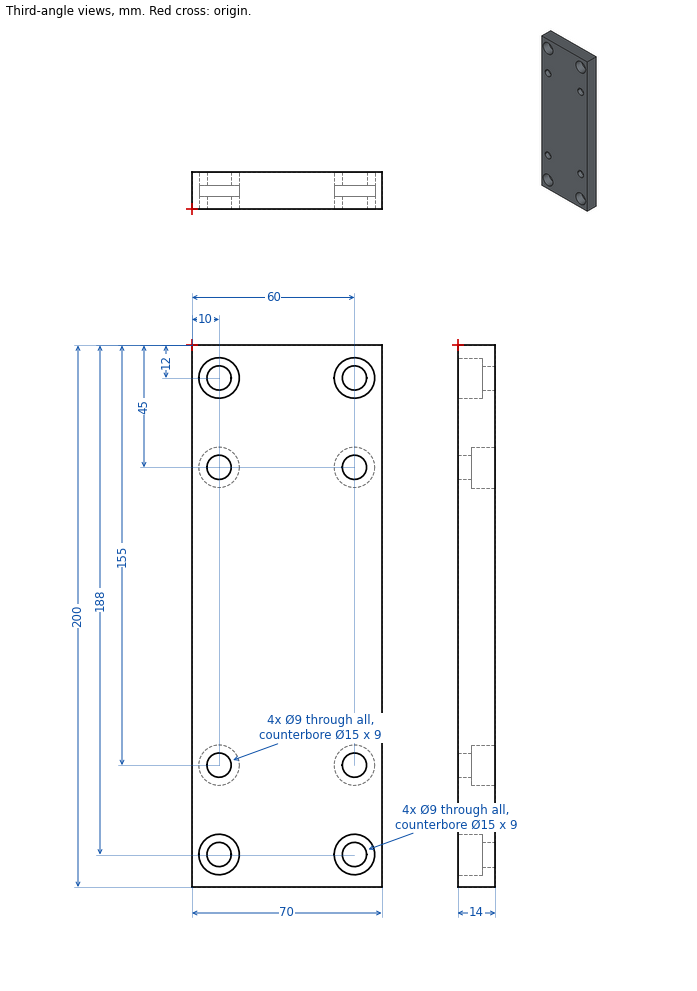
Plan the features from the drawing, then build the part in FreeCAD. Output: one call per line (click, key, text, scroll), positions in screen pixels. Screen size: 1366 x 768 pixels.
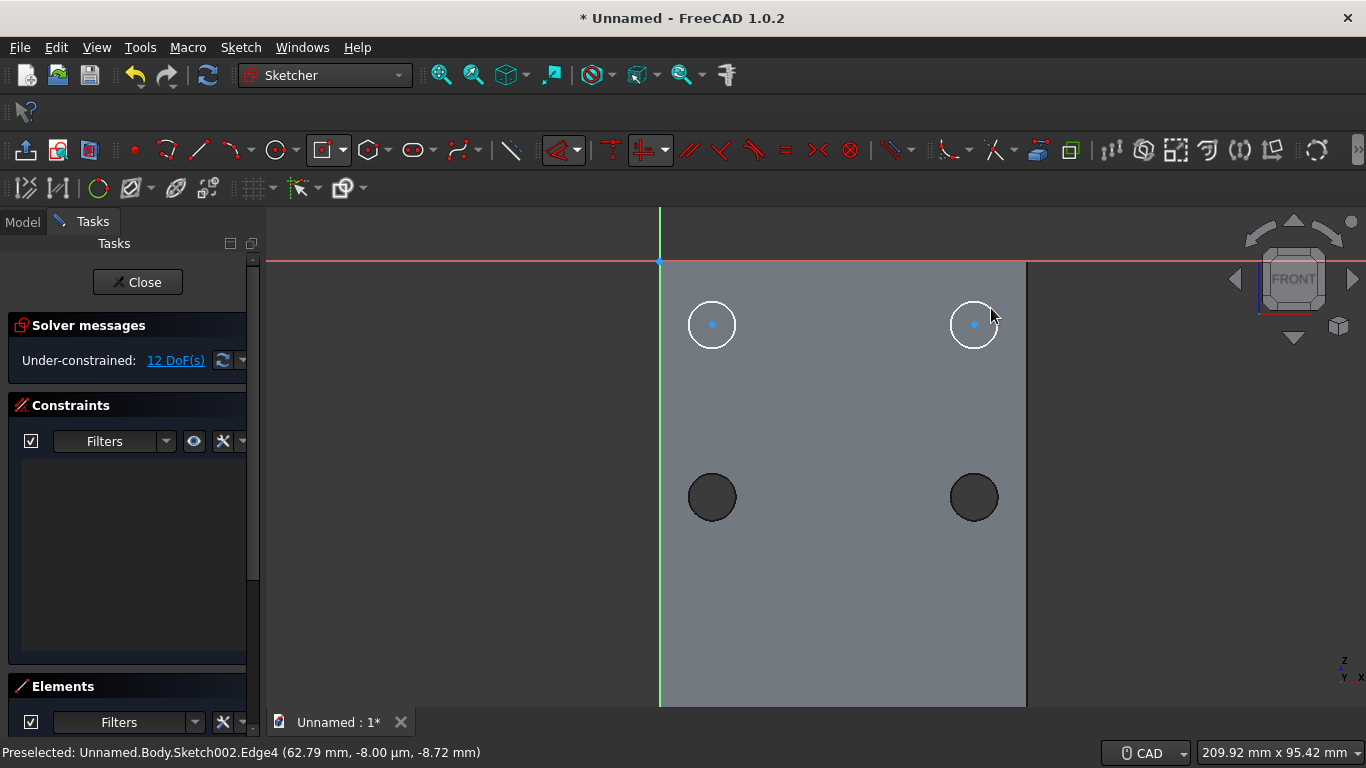
scroll(712, 324, down, 6)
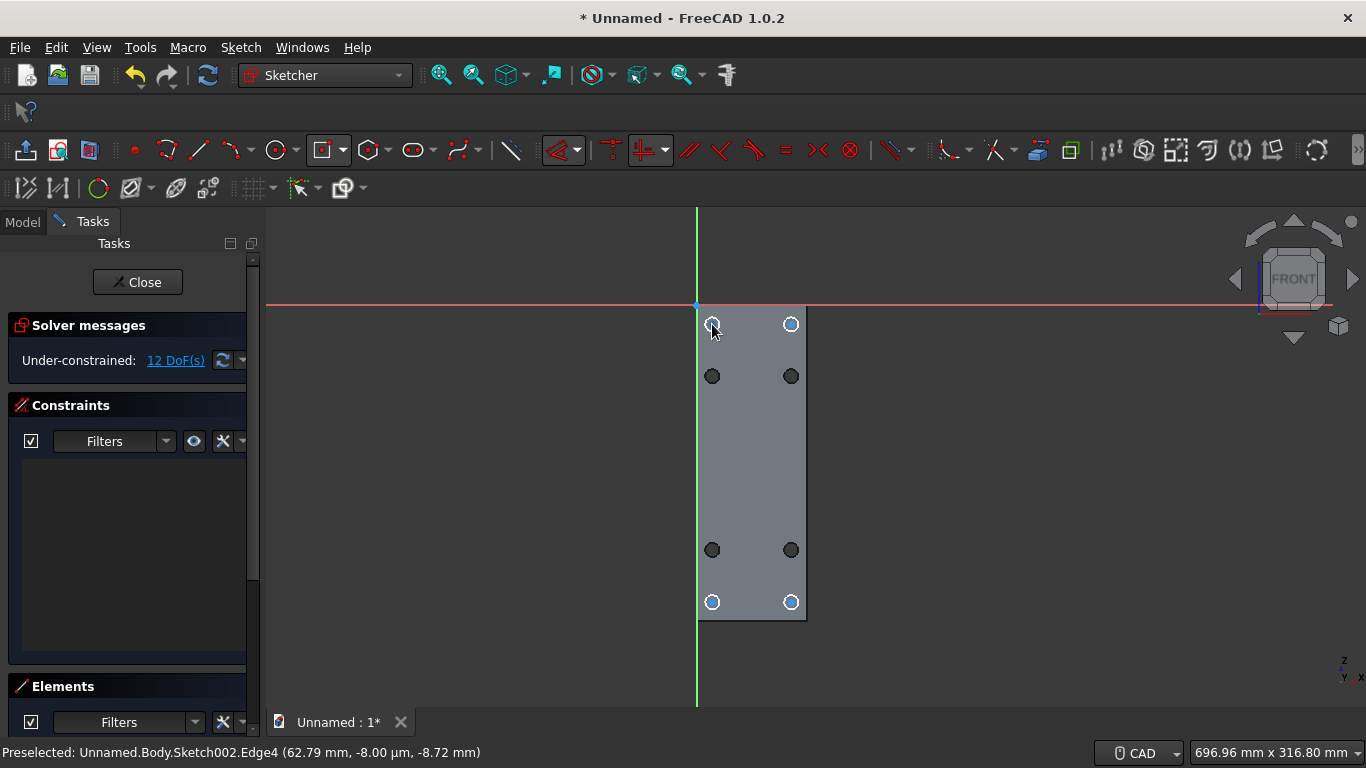
scroll(796, 597, up, 4)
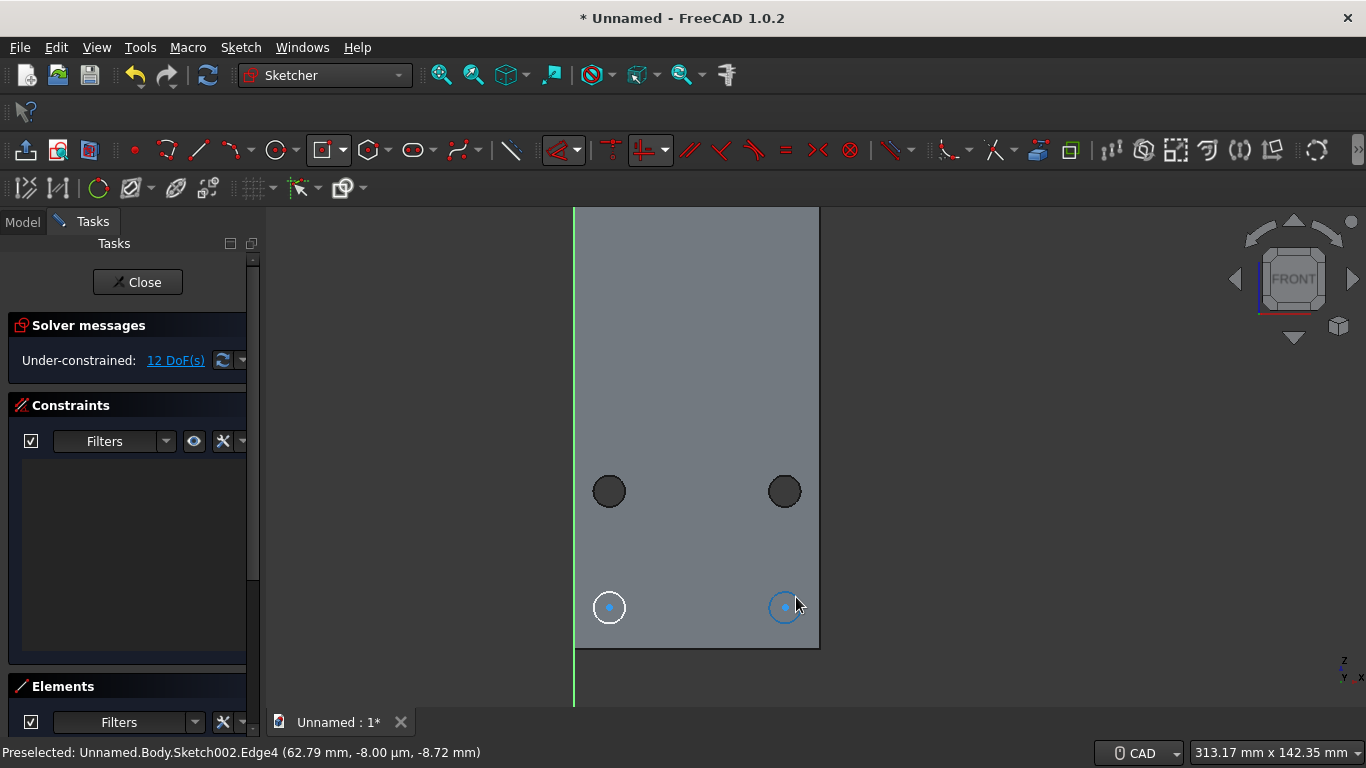
click(796, 597)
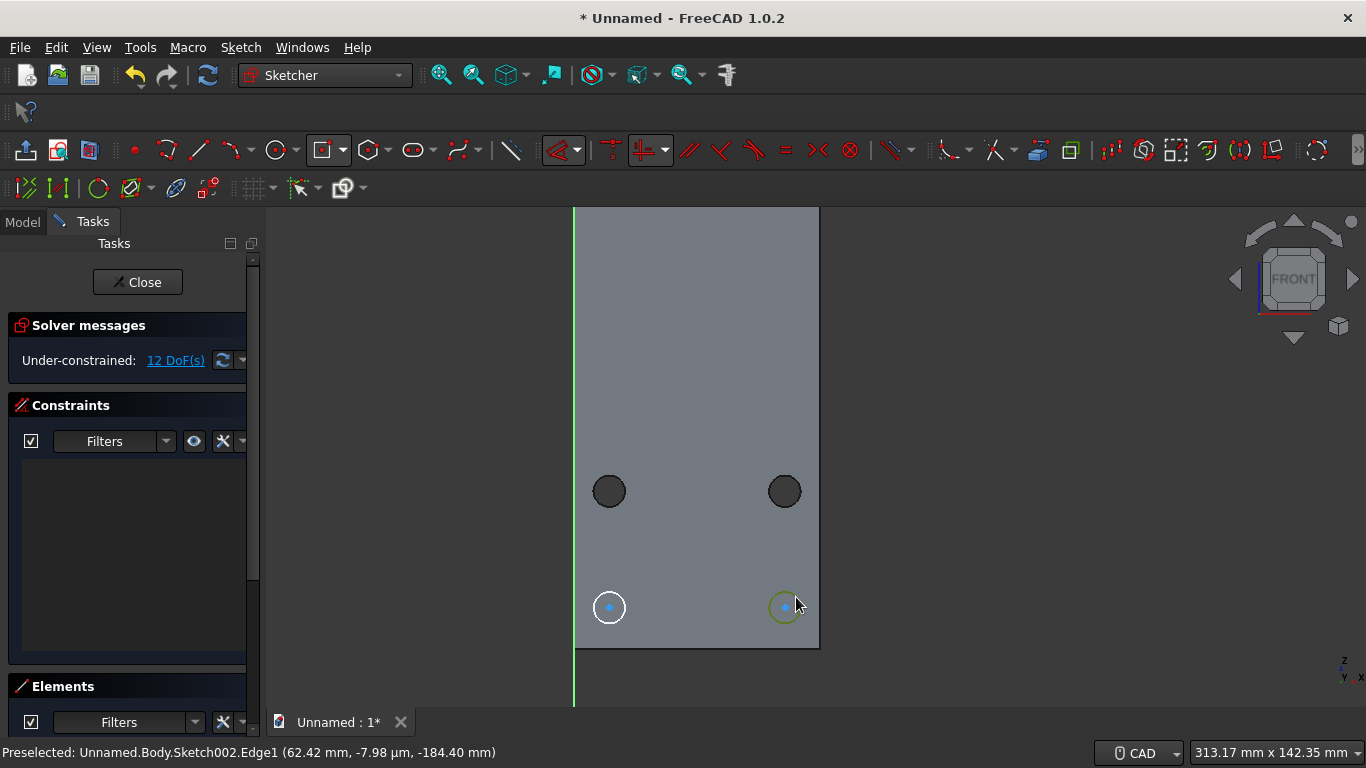
click(620, 597)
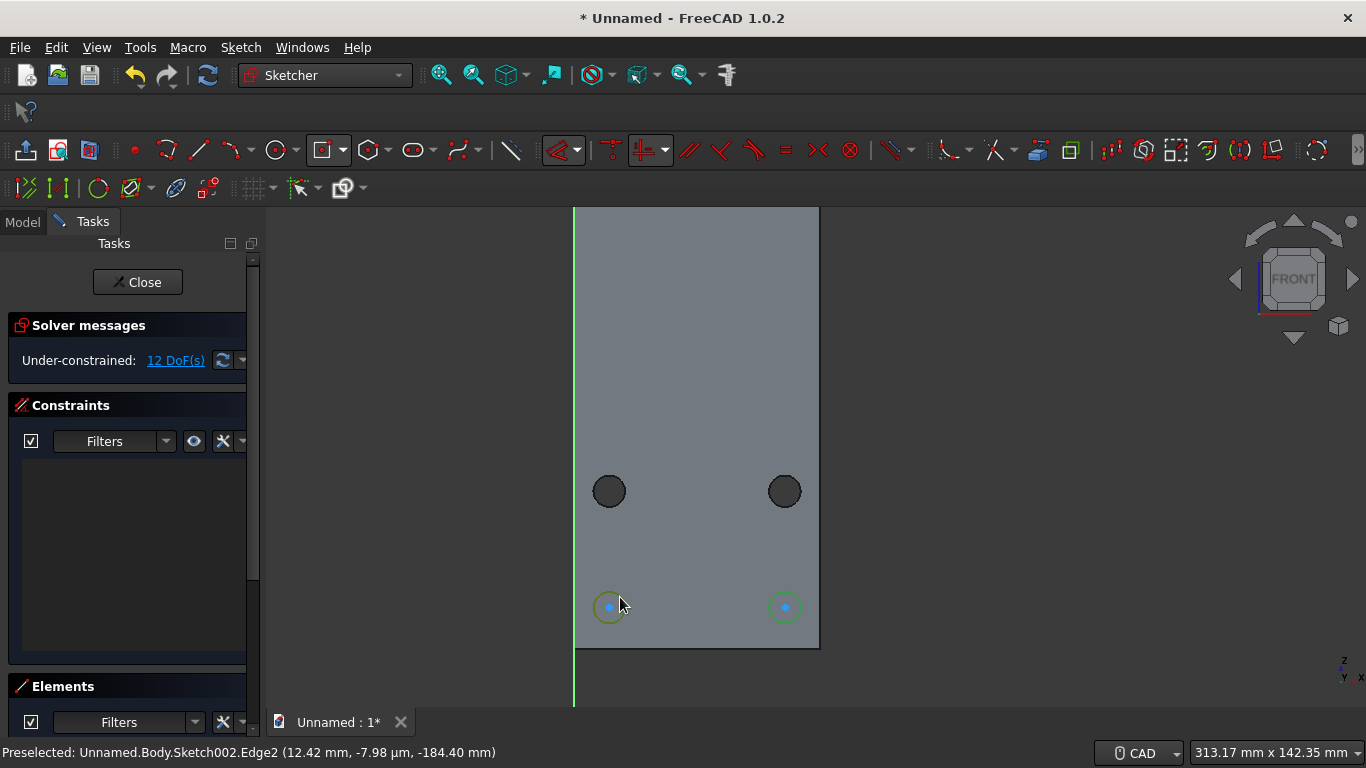
scroll(797, 597, down, 4)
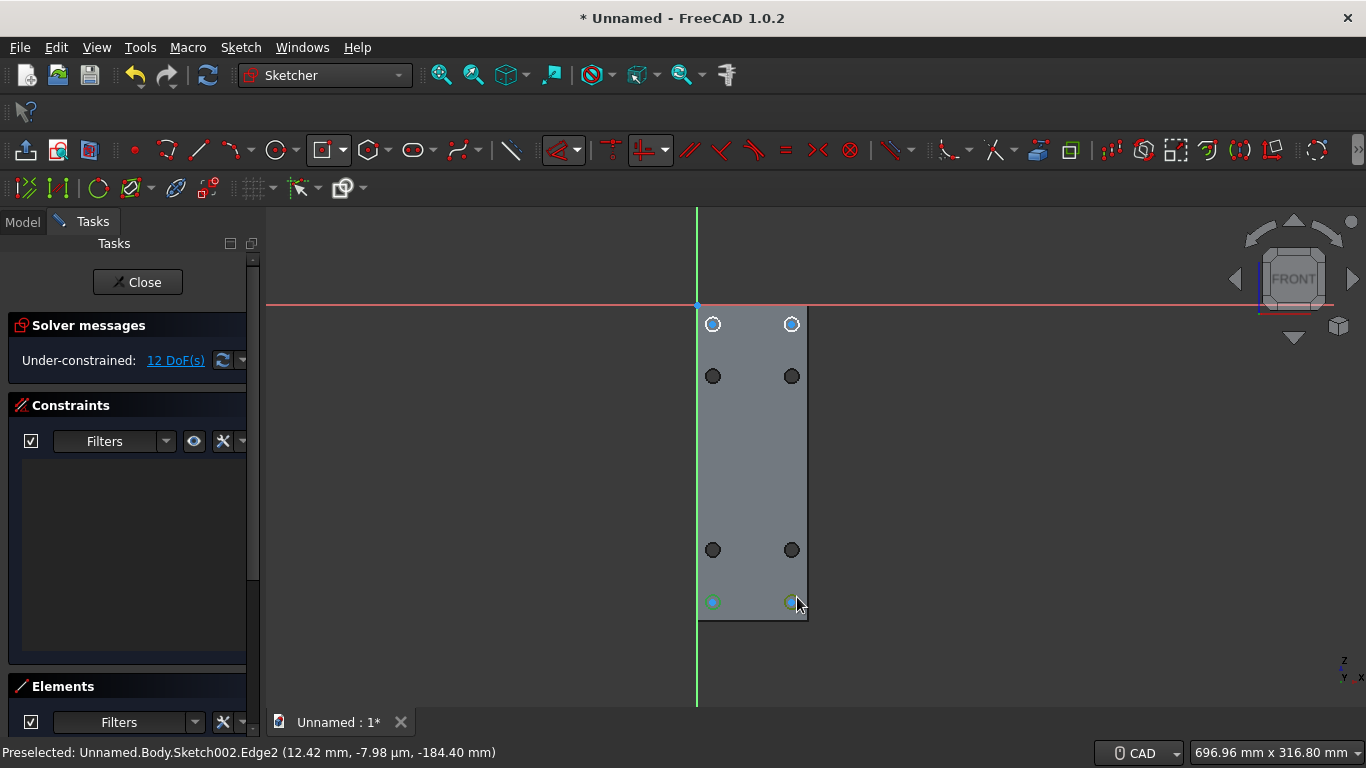
scroll(718, 319, up, 4)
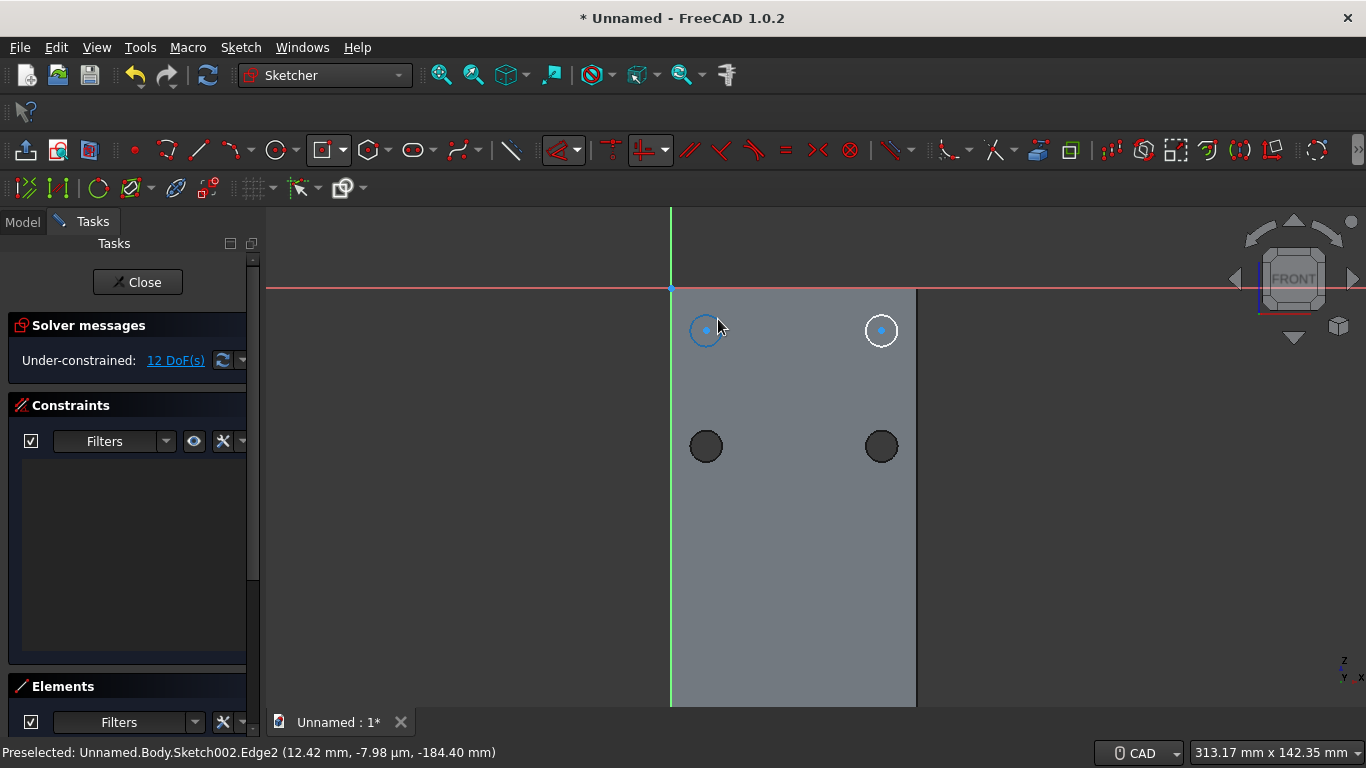
click(717, 320)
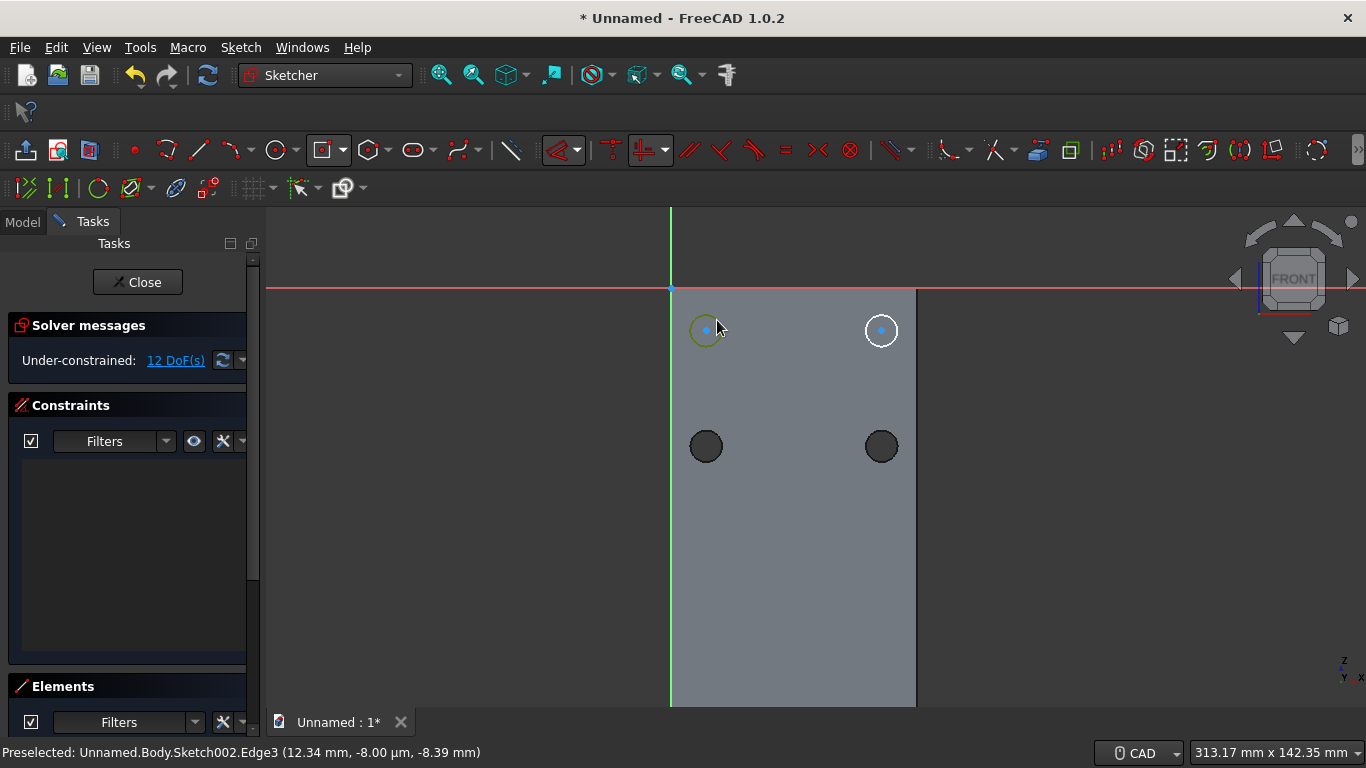
click(893, 320)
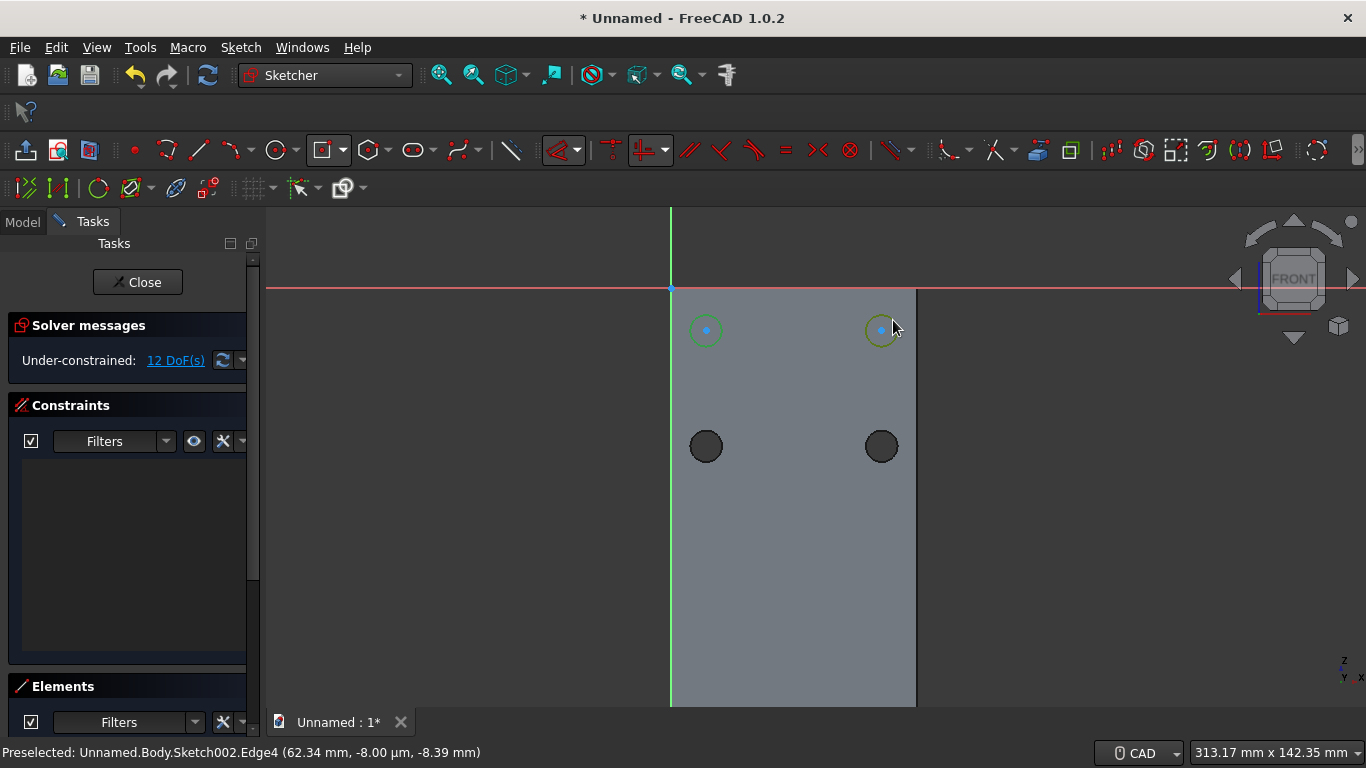
click(786, 150)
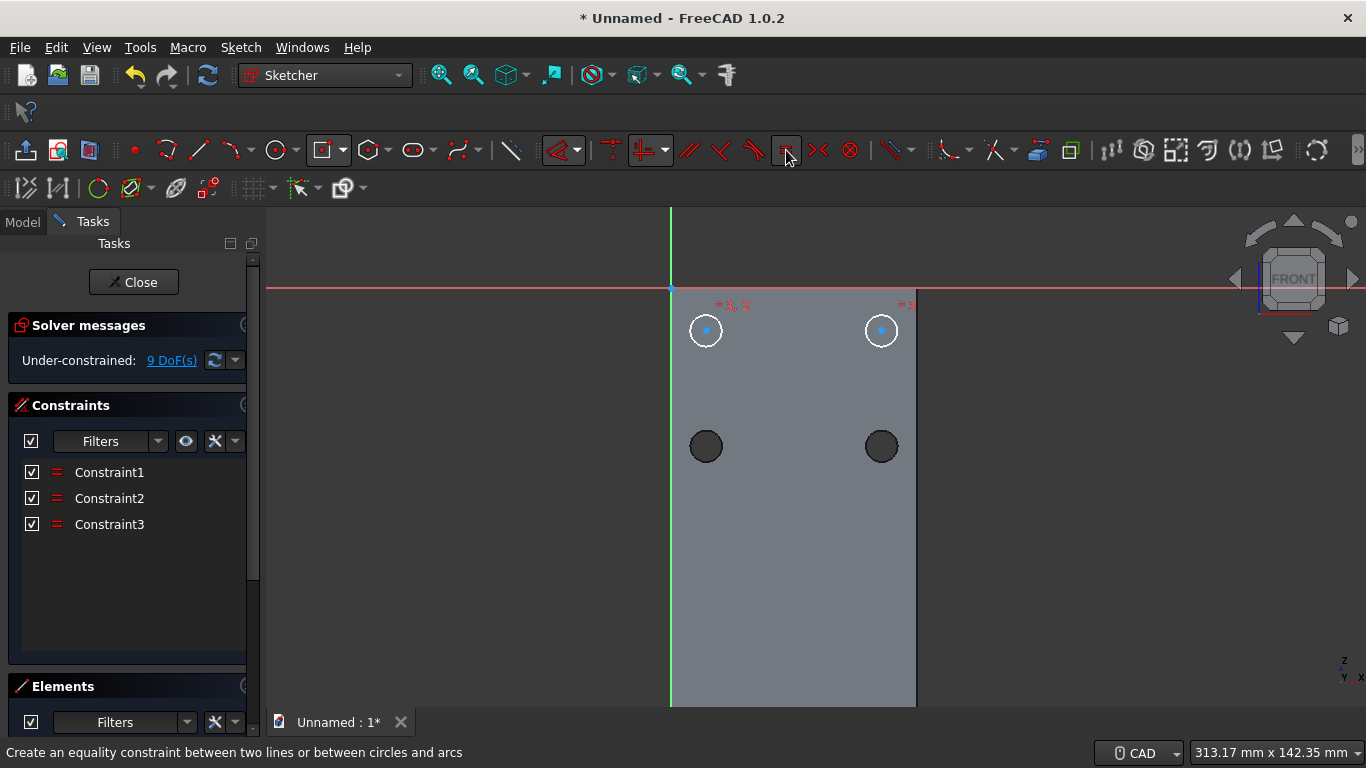
scroll(717, 319, down, 4)